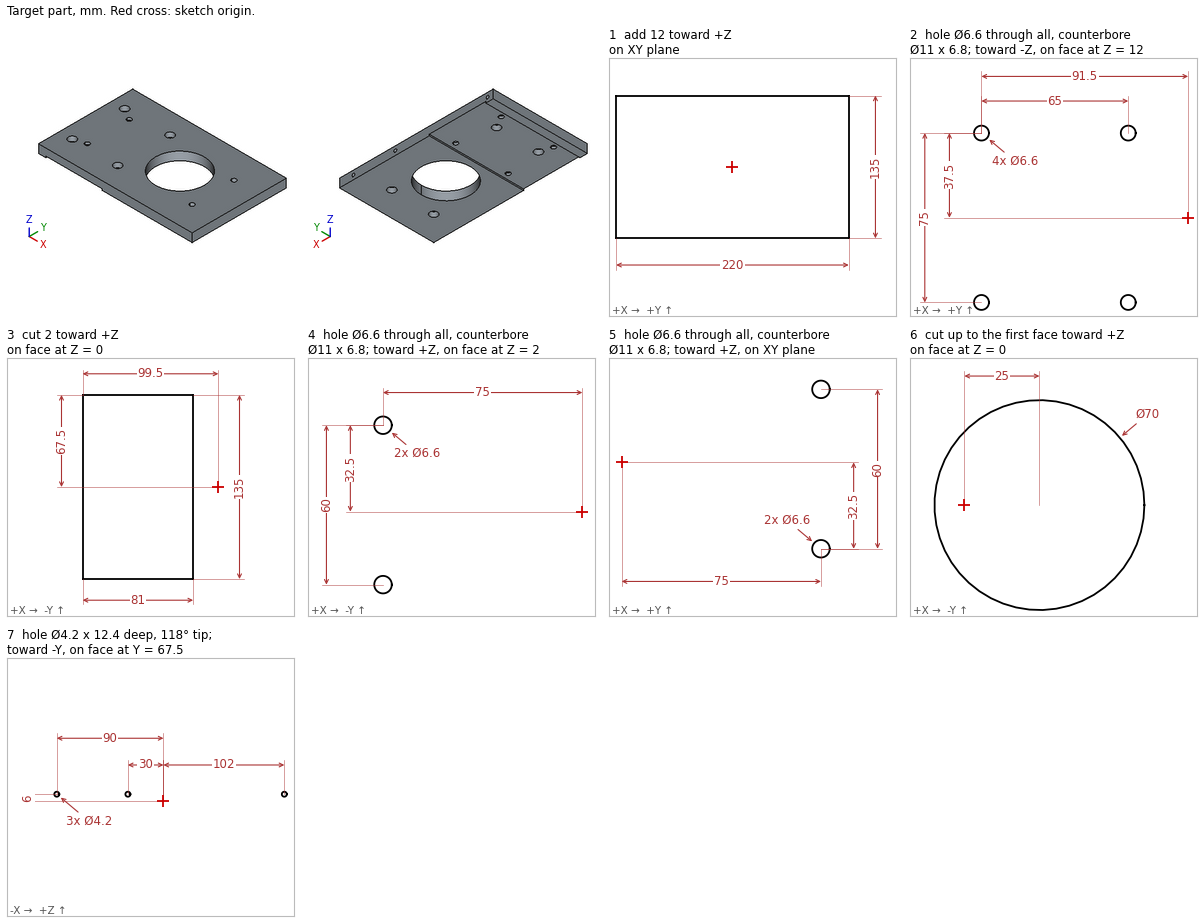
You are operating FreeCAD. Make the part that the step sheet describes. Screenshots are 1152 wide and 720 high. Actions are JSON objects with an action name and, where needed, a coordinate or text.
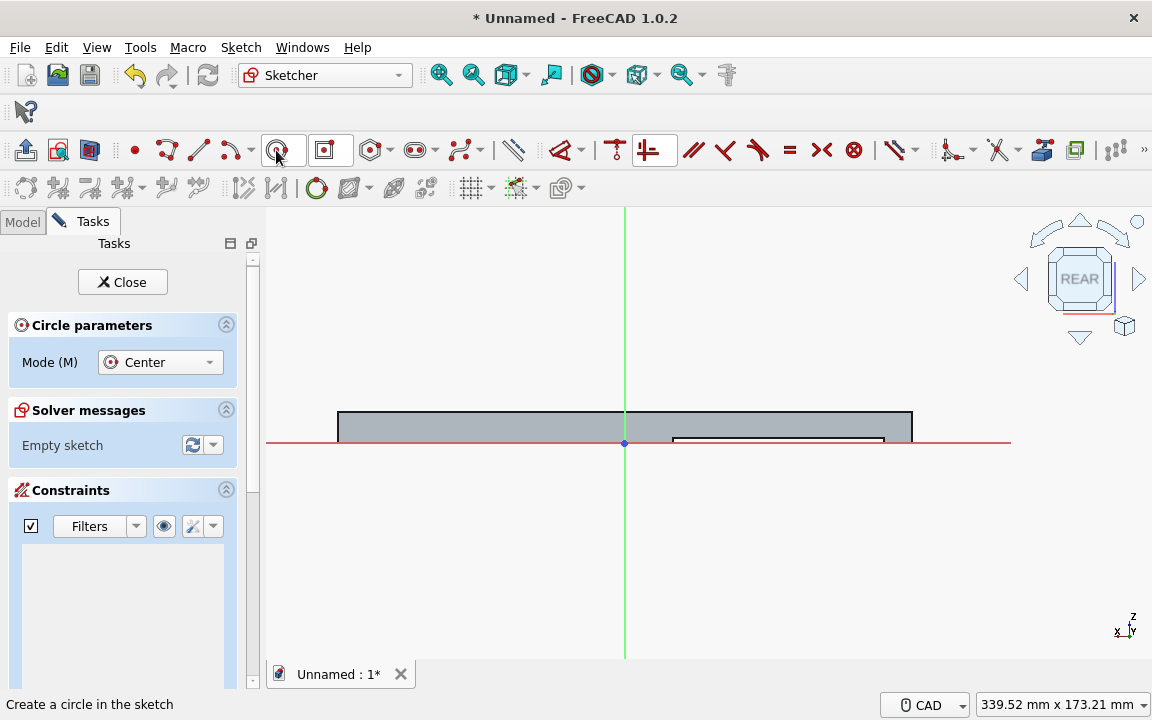
{"action": "scroll", "coordinate": [390, 428], "scroll_direction": "up", "scroll_amount": 8}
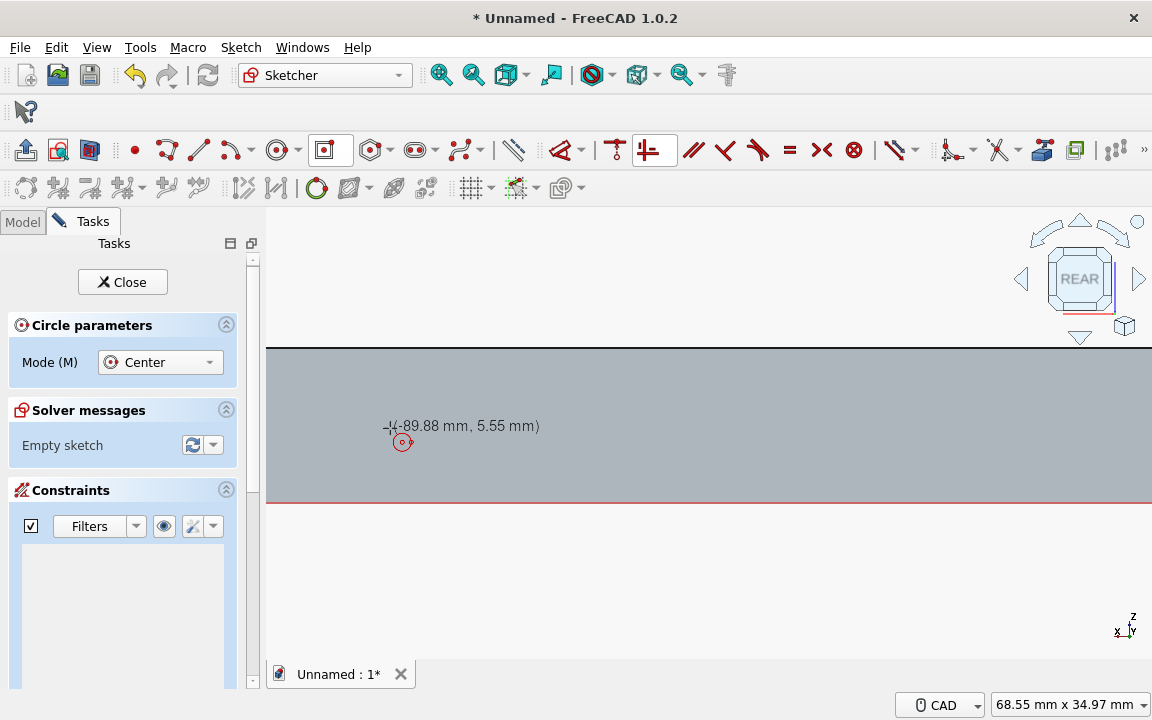
{"action": "scroll", "coordinate": [390, 429], "scroll_direction": "down", "scroll_amount": 8}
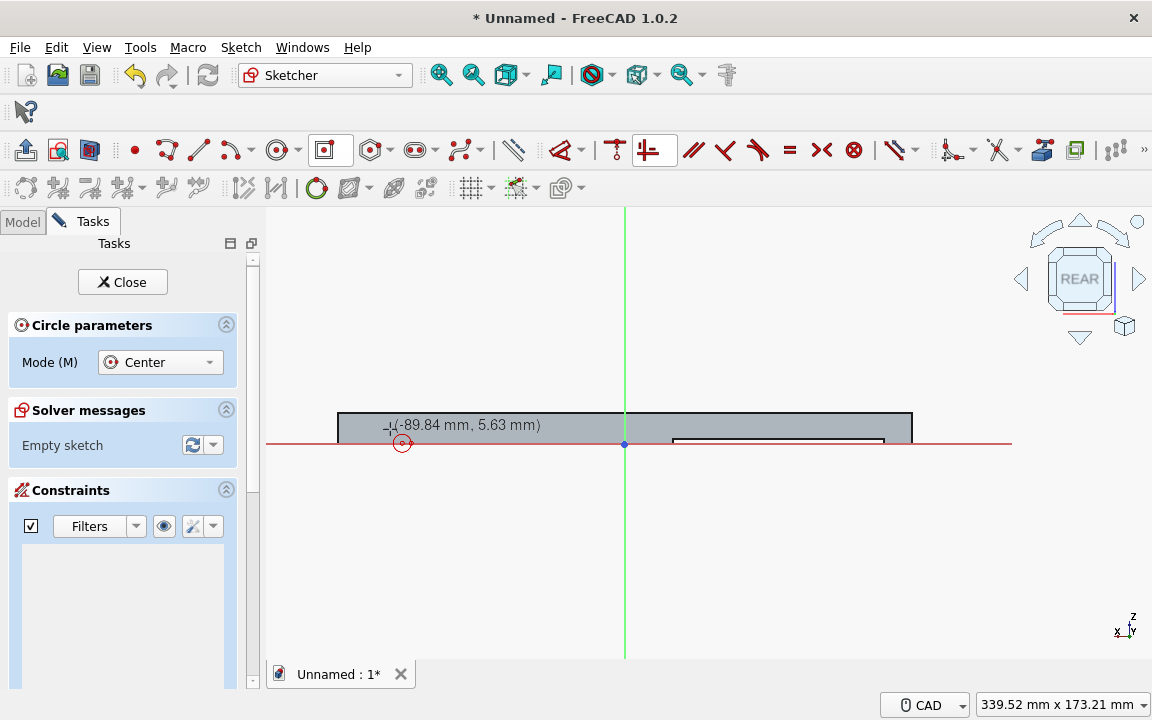
{"action": "left_click", "coordinate": [390, 429]}
{"action": "mouse_move", "coordinate": [394, 425]}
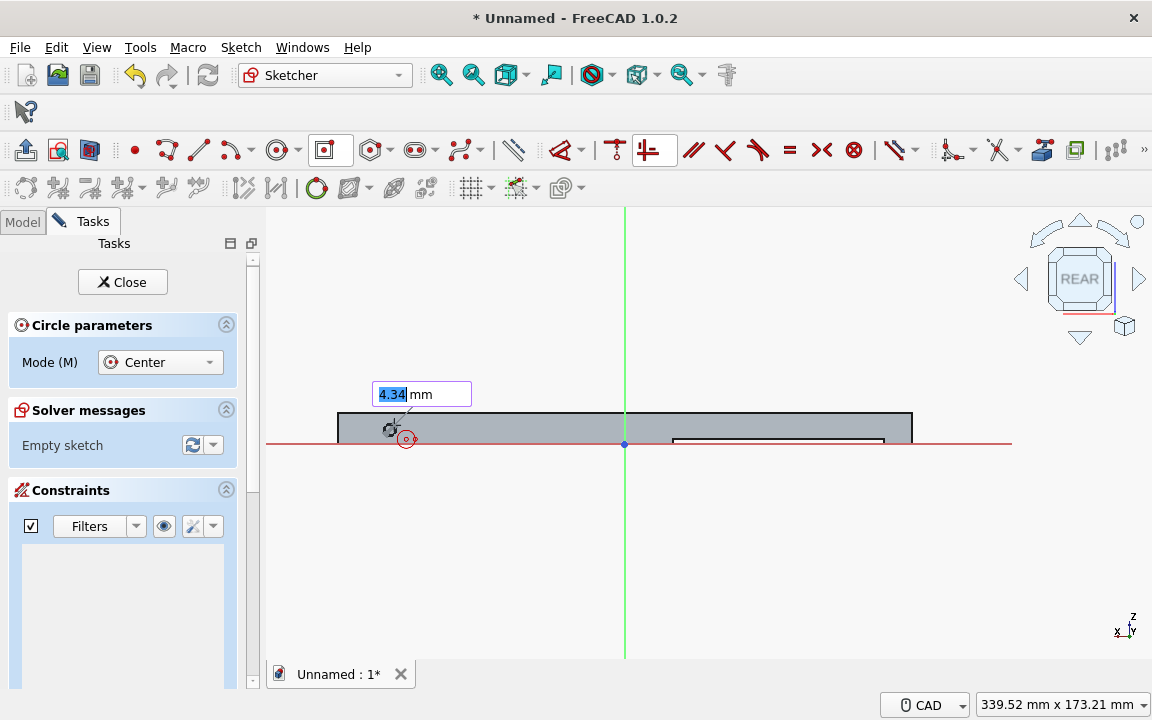
{"action": "type", "text": "4.2"}
{"action": "key", "text": "Return"}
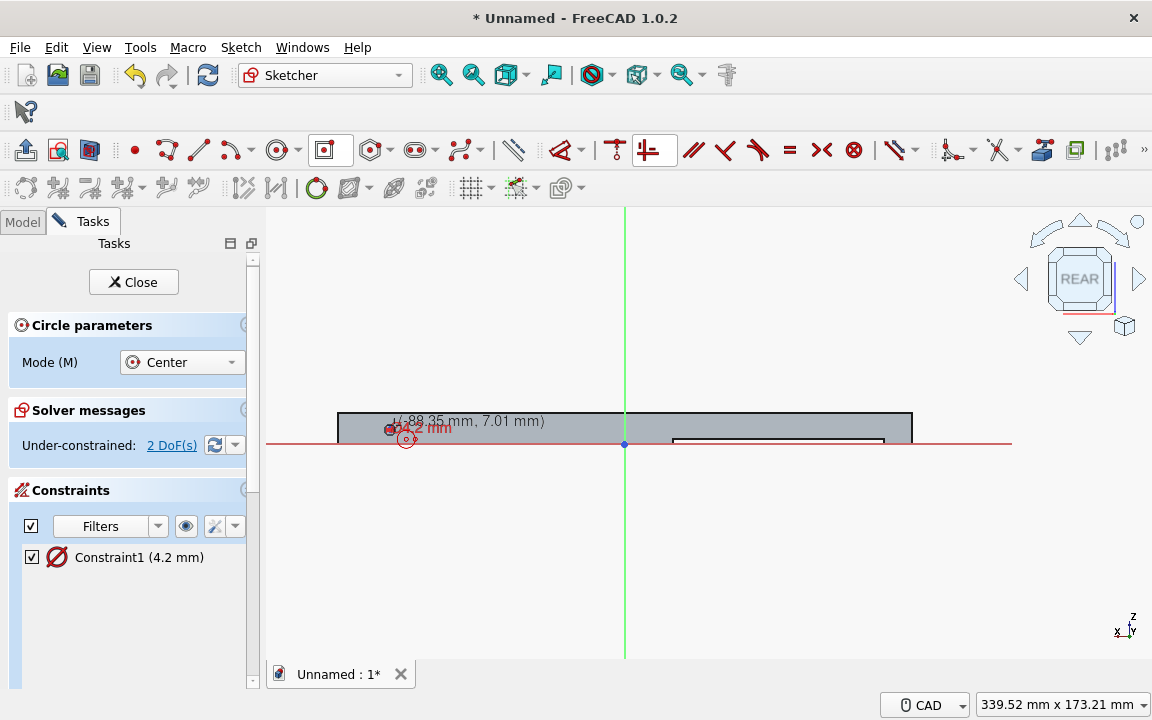
{"action": "scroll", "coordinate": [546, 429], "scroll_direction": "up", "scroll_amount": 8}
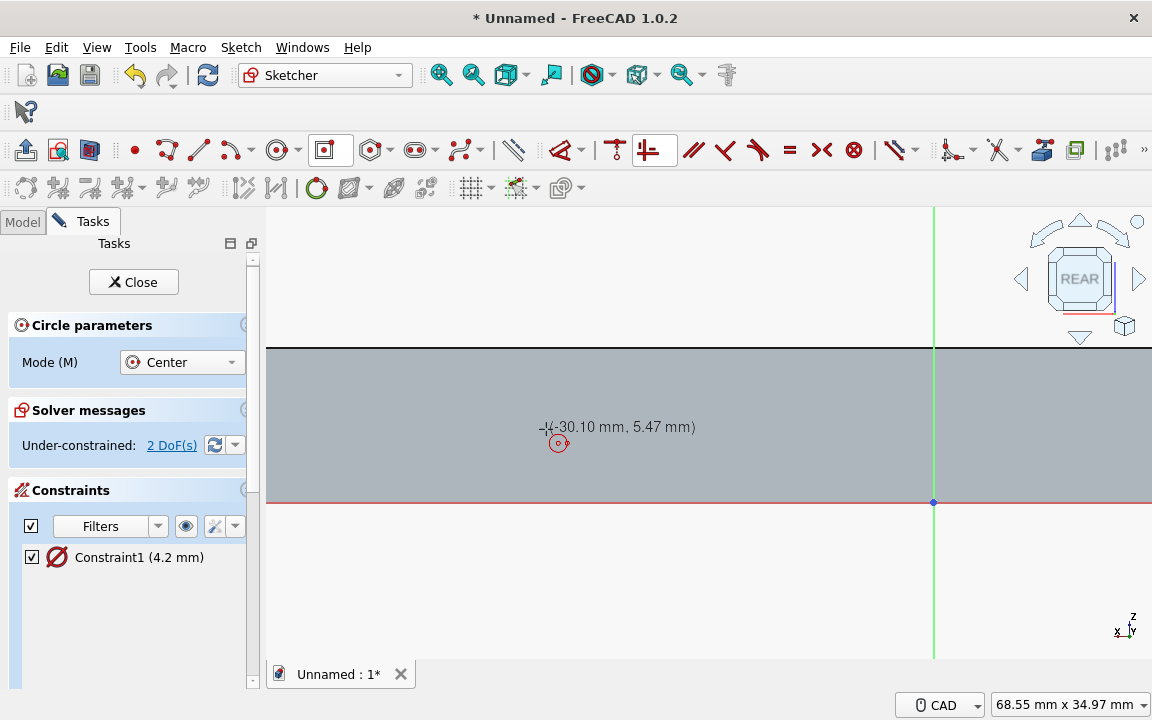
{"action": "scroll", "coordinate": [547, 429], "scroll_direction": "down", "scroll_amount": 8}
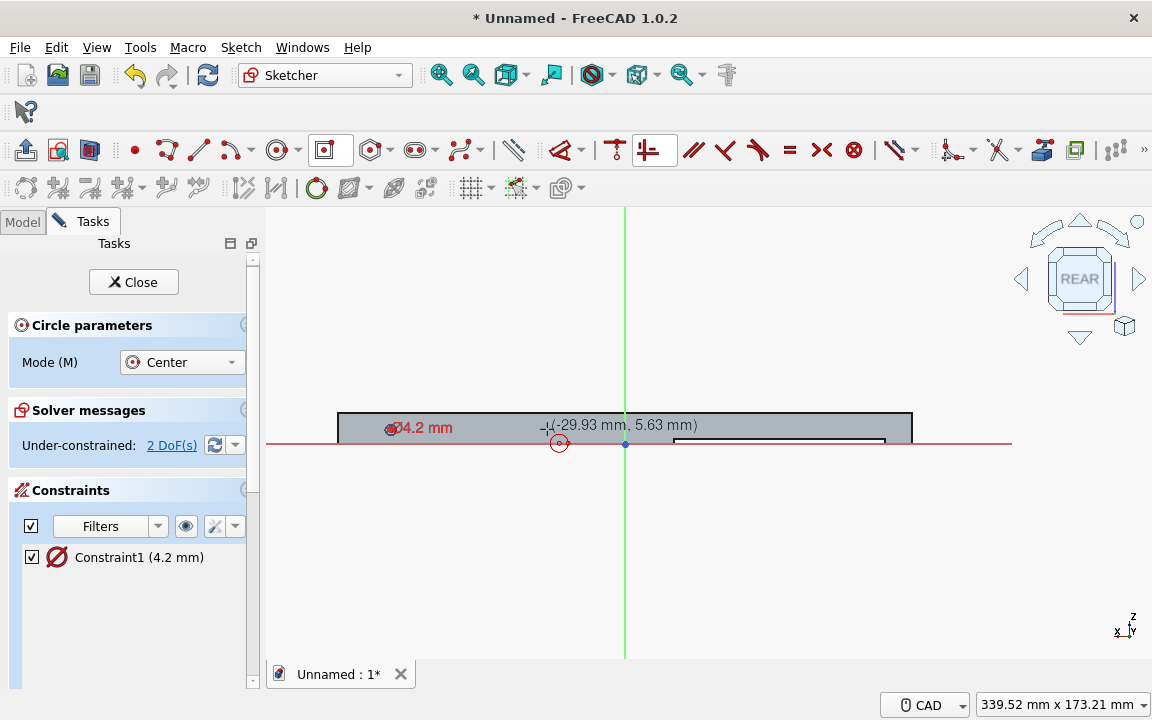
{"action": "left_click", "coordinate": [547, 429]}
{"action": "mouse_move", "coordinate": [551, 425]}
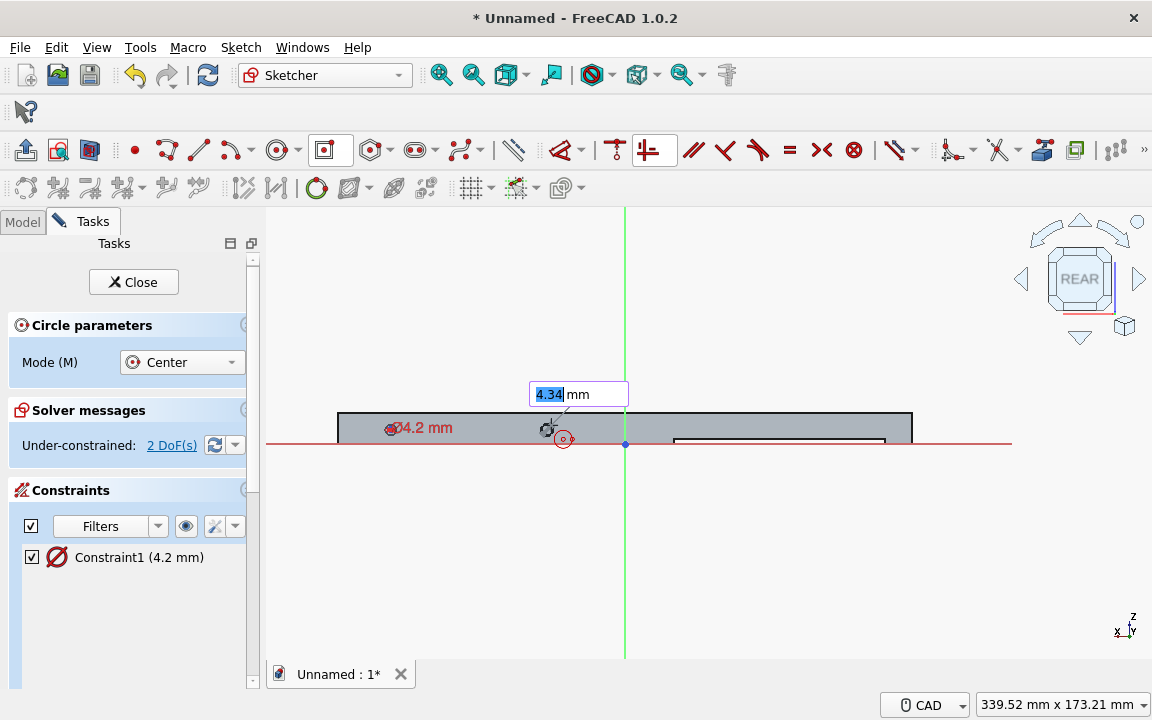
{"action": "type", "text": "4.2"}
{"action": "key", "text": "Return"}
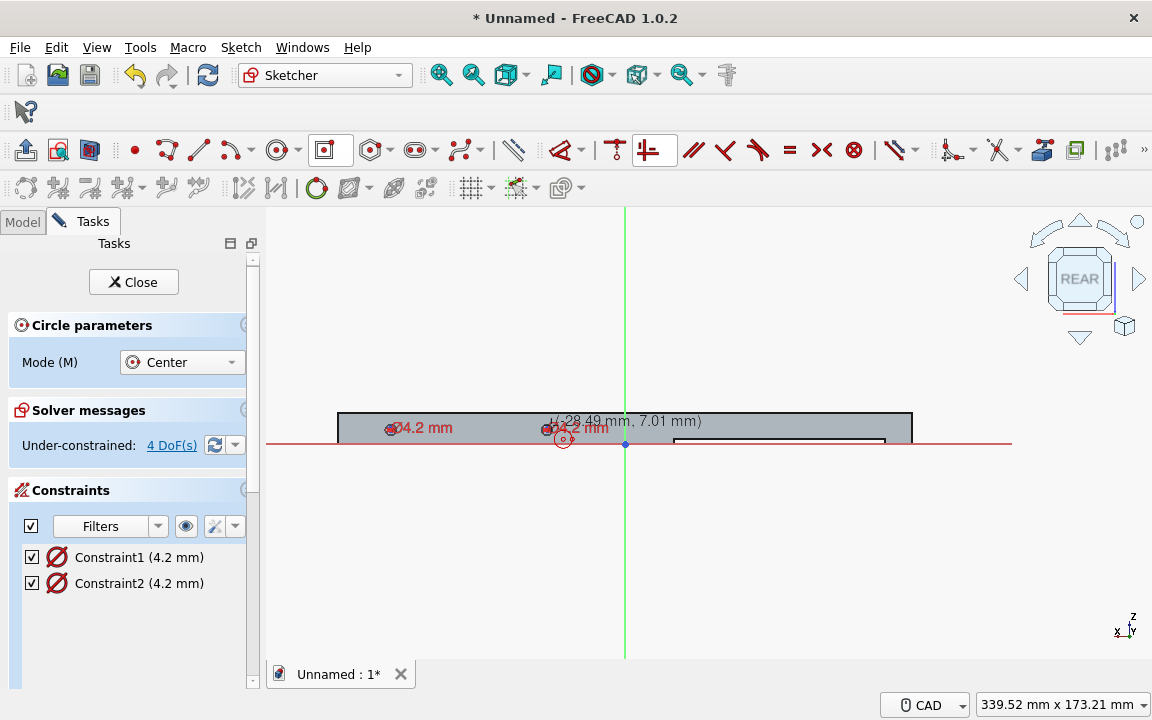
{"action": "scroll", "coordinate": [892, 429], "scroll_direction": "up", "scroll_amount": 8}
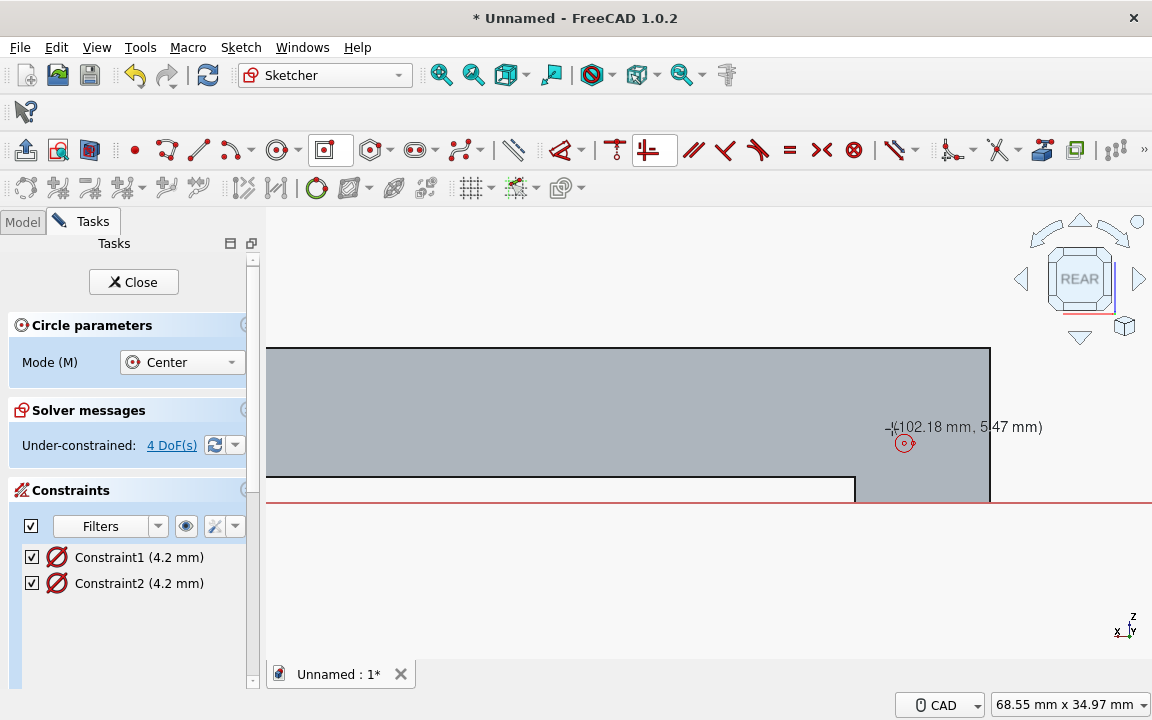
{"action": "scroll", "coordinate": [892, 429], "scroll_direction": "down", "scroll_amount": 8}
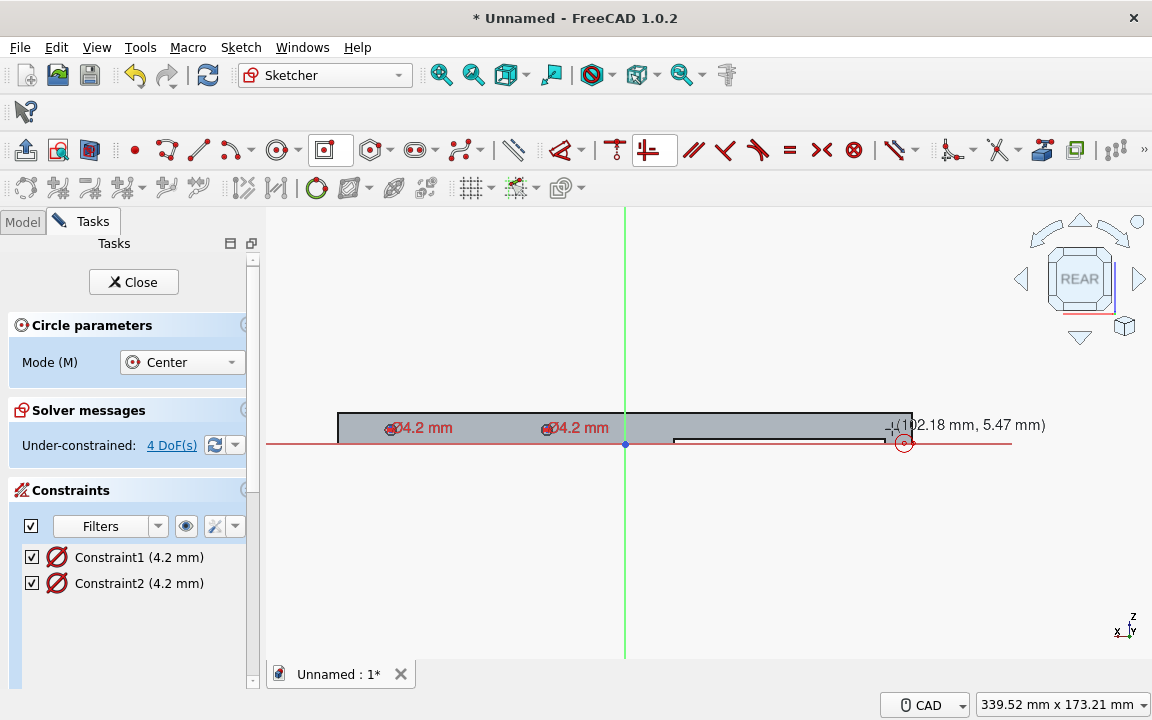
{"action": "left_click", "coordinate": [892, 429]}
{"action": "mouse_move", "coordinate": [895, 425]}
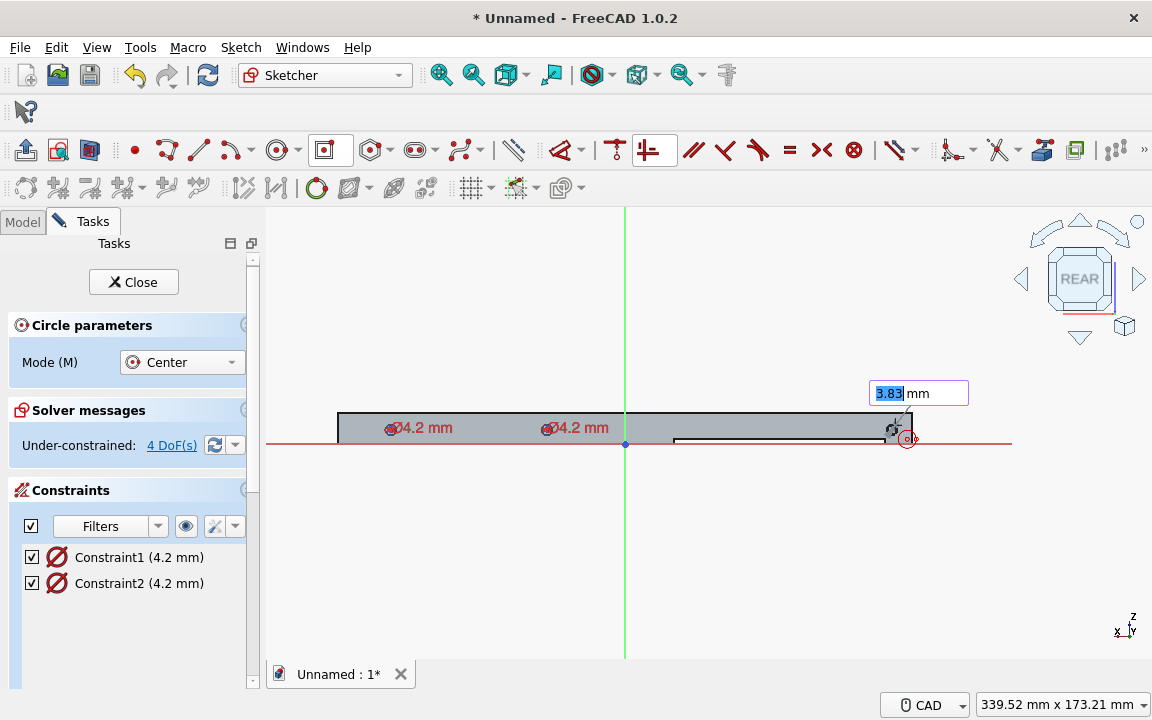
{"action": "type", "text": "4.2"}
{"action": "key", "text": "Return"}
{"action": "key", "text": "Escape"}